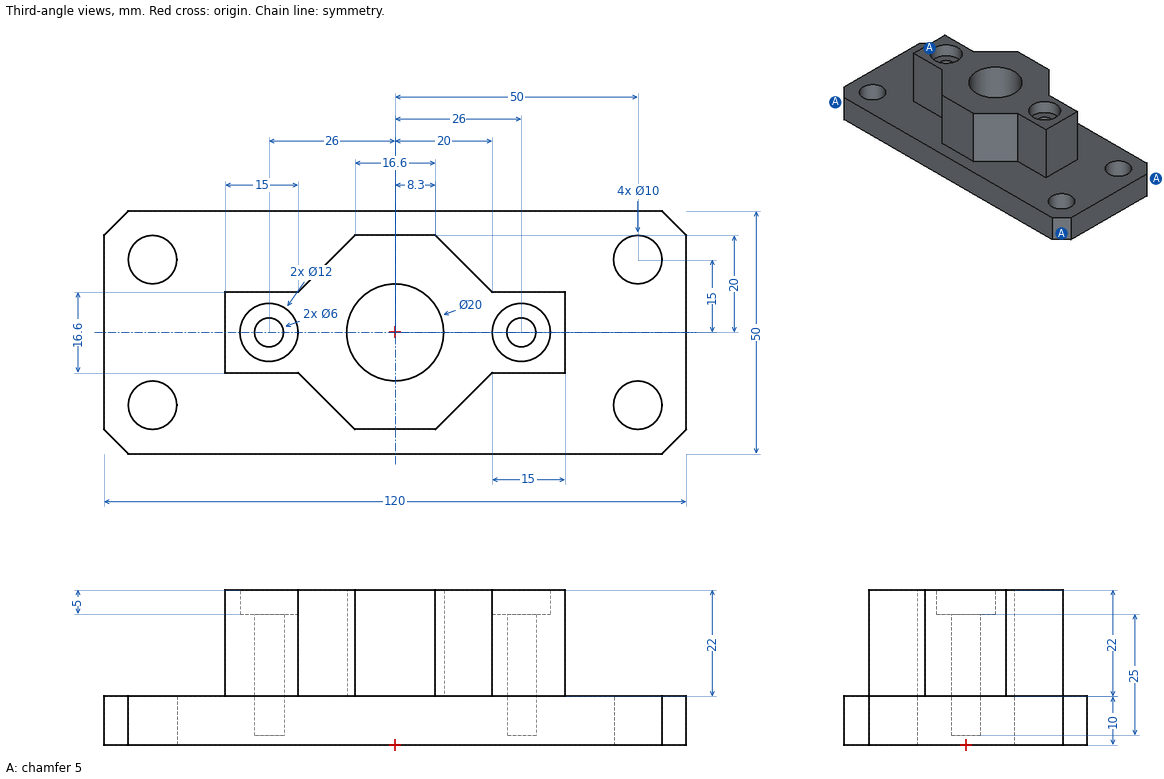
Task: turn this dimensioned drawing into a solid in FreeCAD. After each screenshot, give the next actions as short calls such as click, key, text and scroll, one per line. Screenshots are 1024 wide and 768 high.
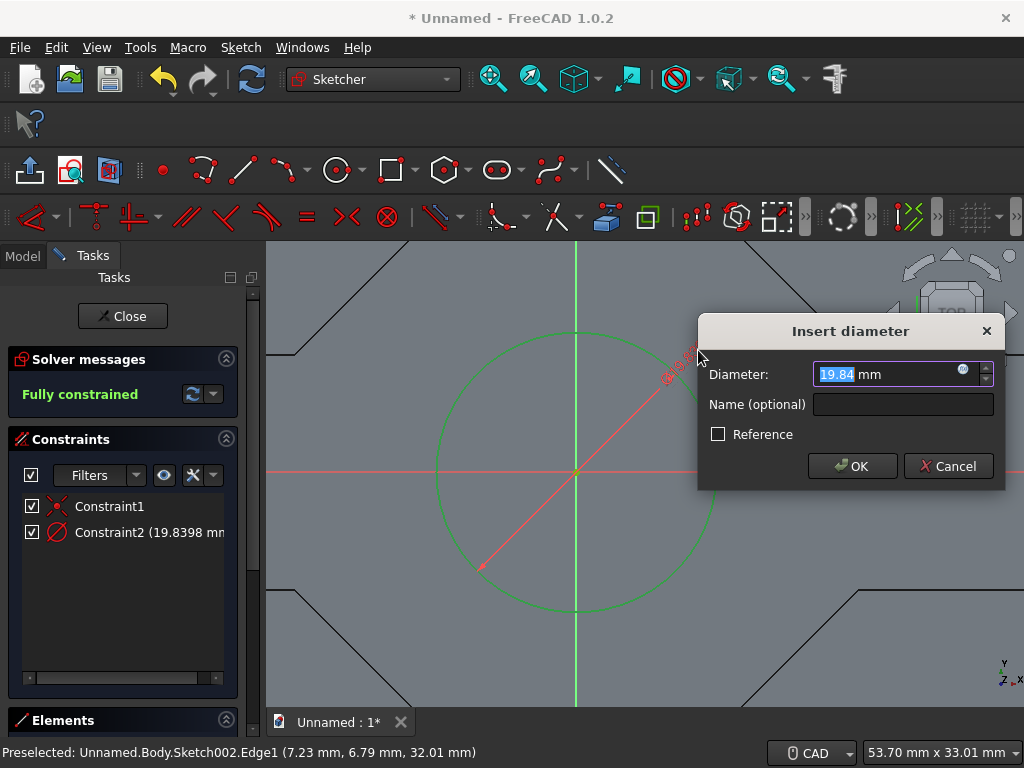
text(20)
key(Return)
key(Escape)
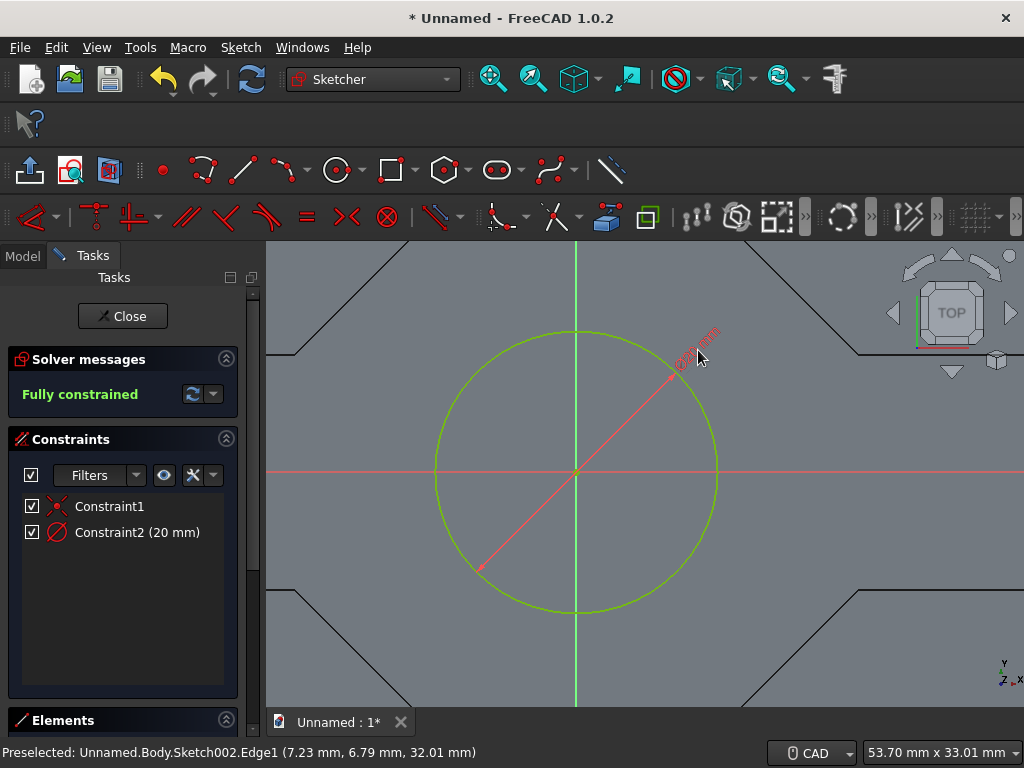
click(123, 316)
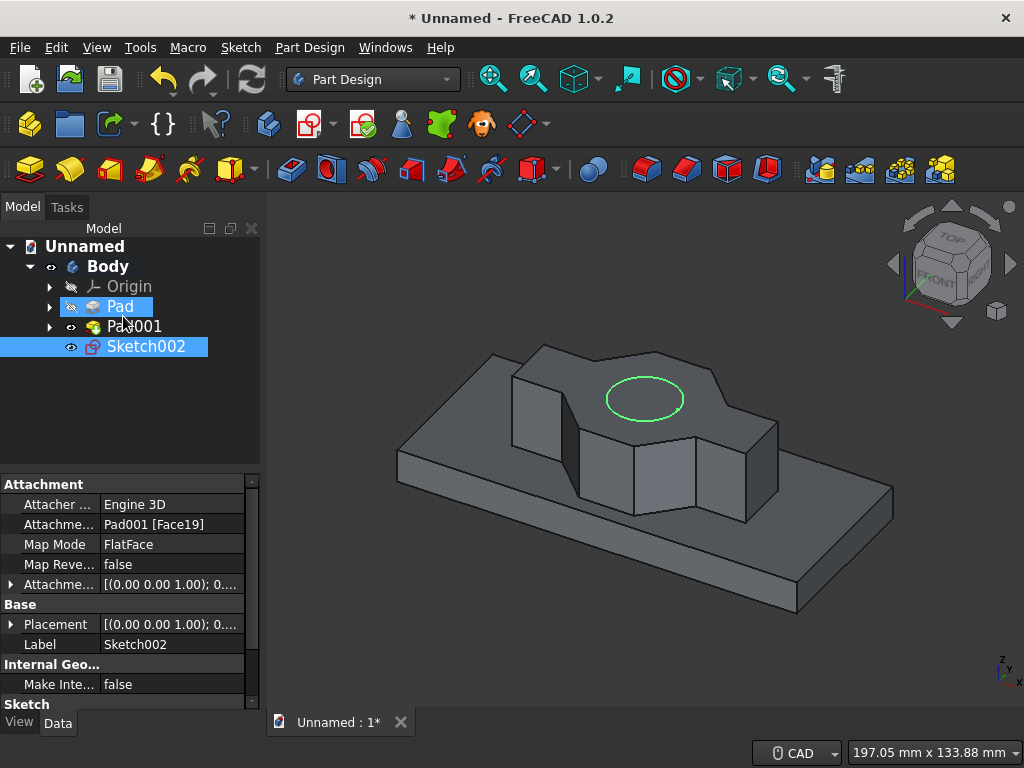
click(292, 170)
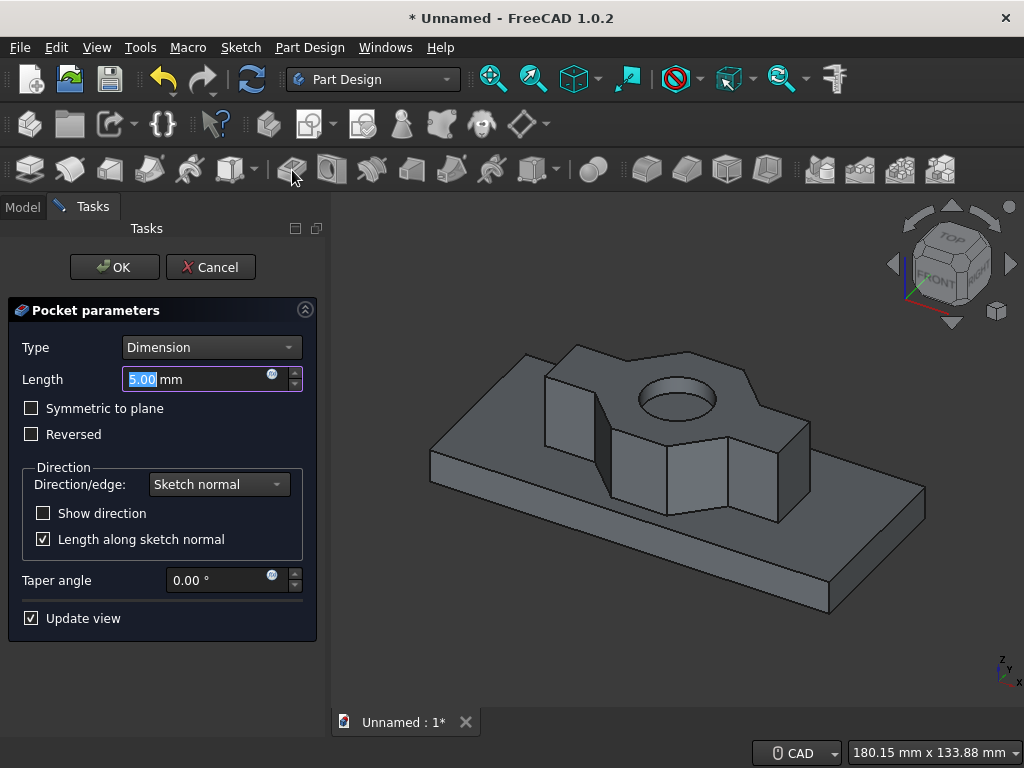
text(22)
key(Tab)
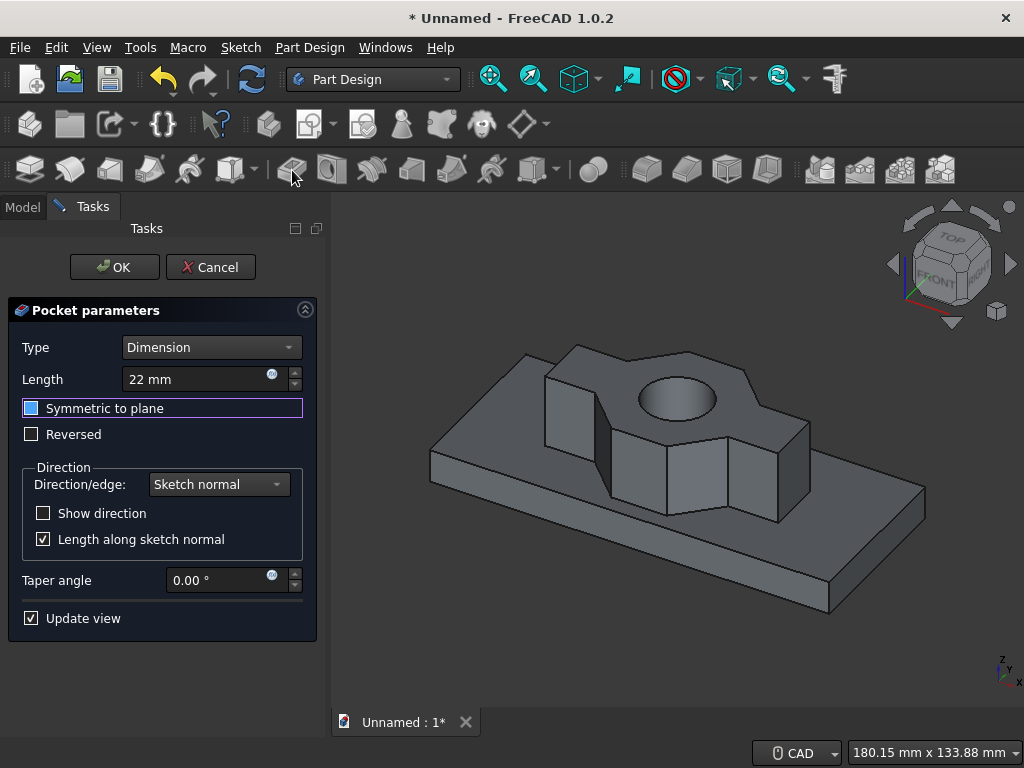
click(115, 267)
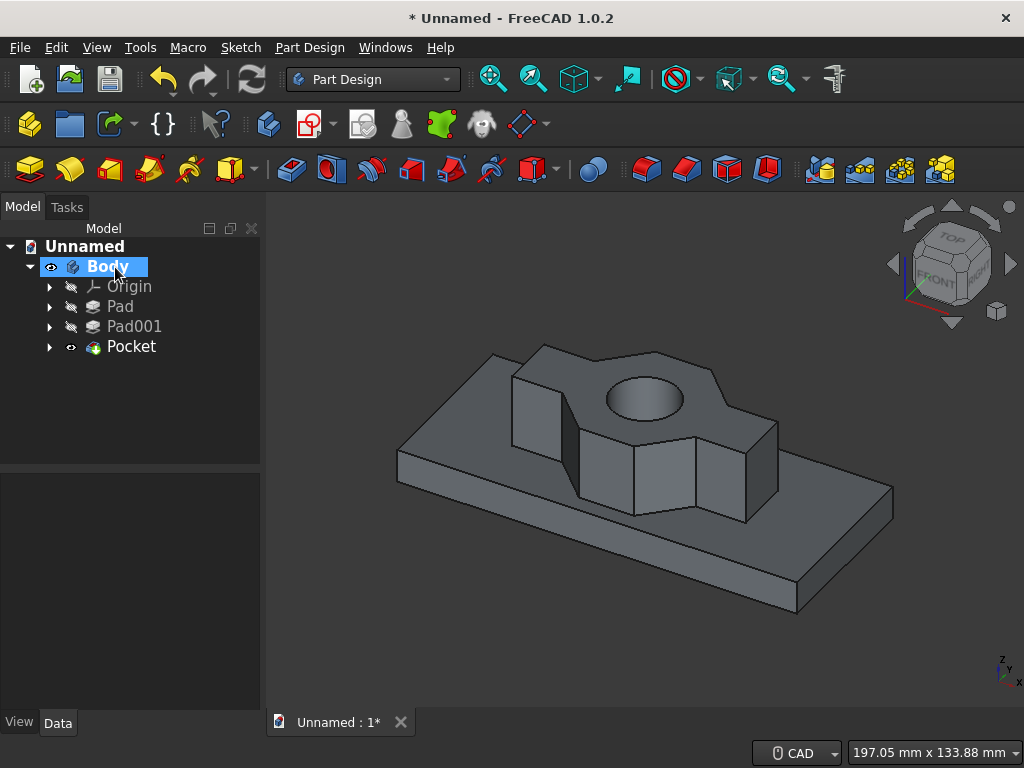
click(712, 420)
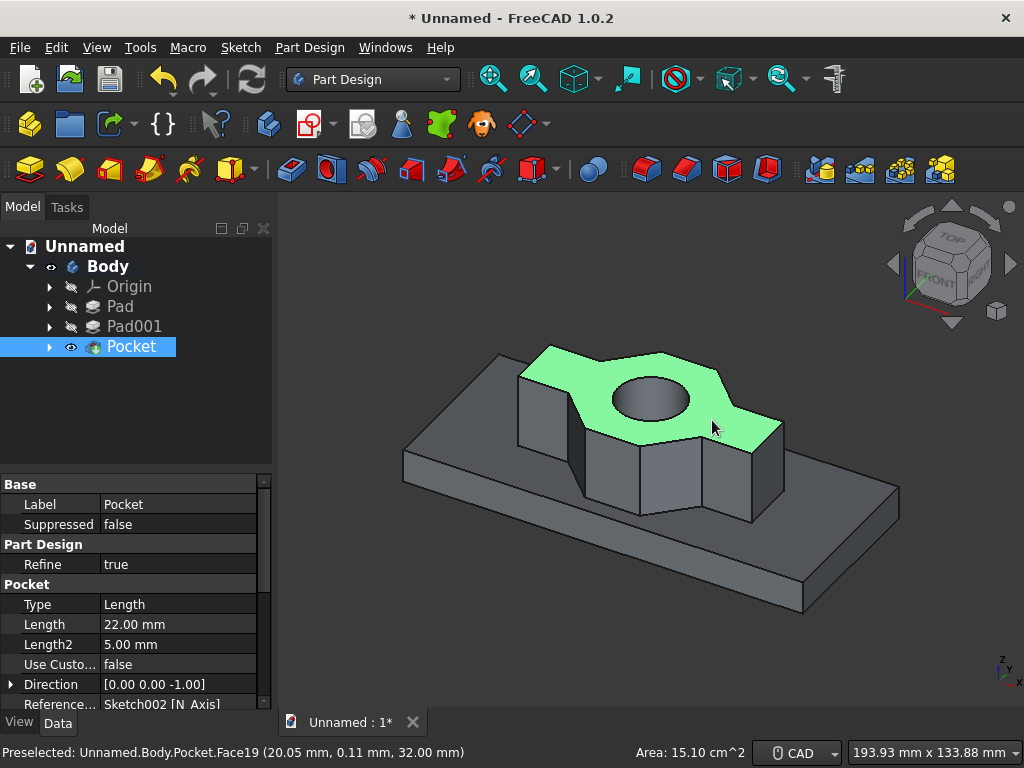
click(310, 124)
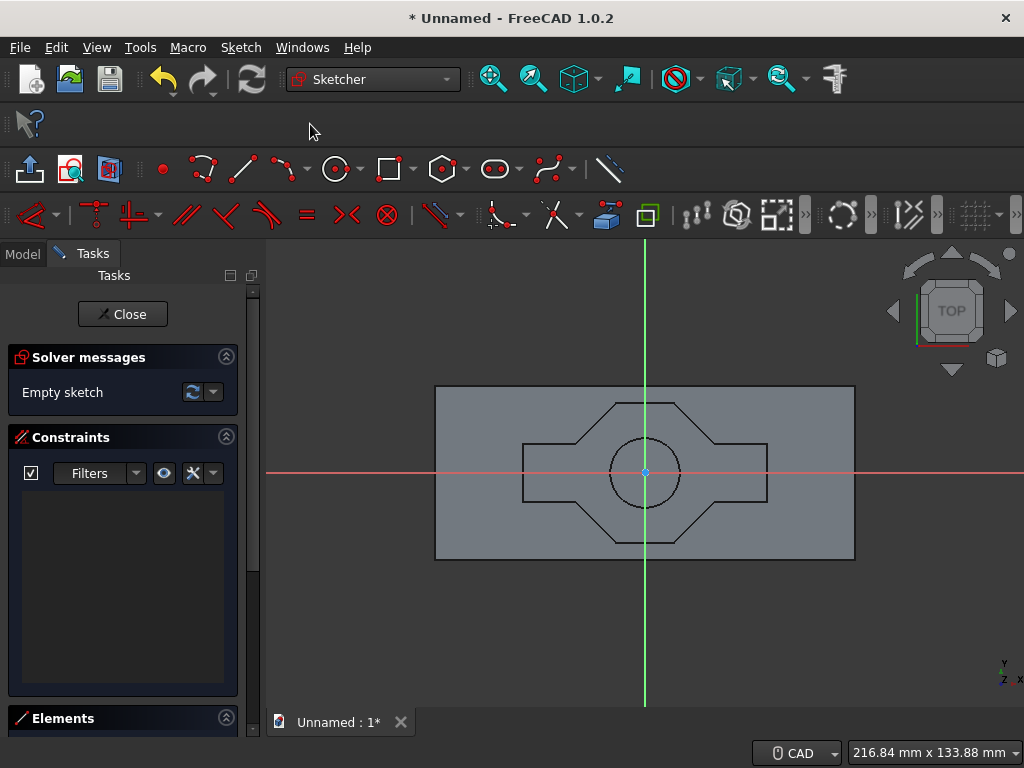
scroll(728, 473, up, 3)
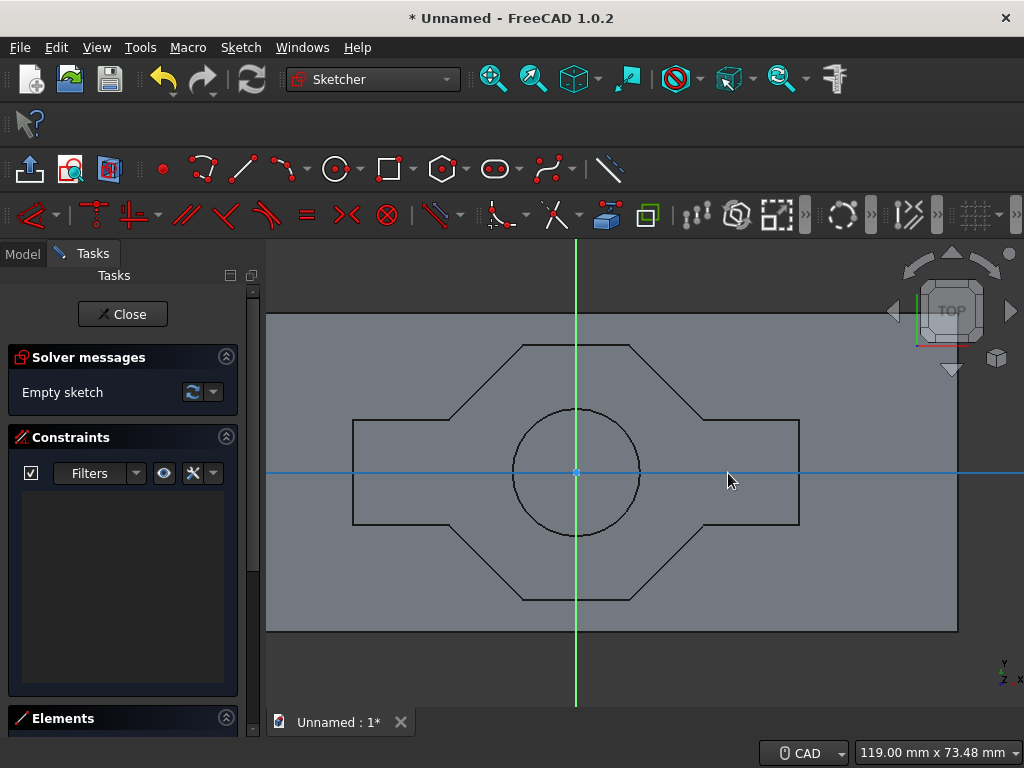
click(336, 170)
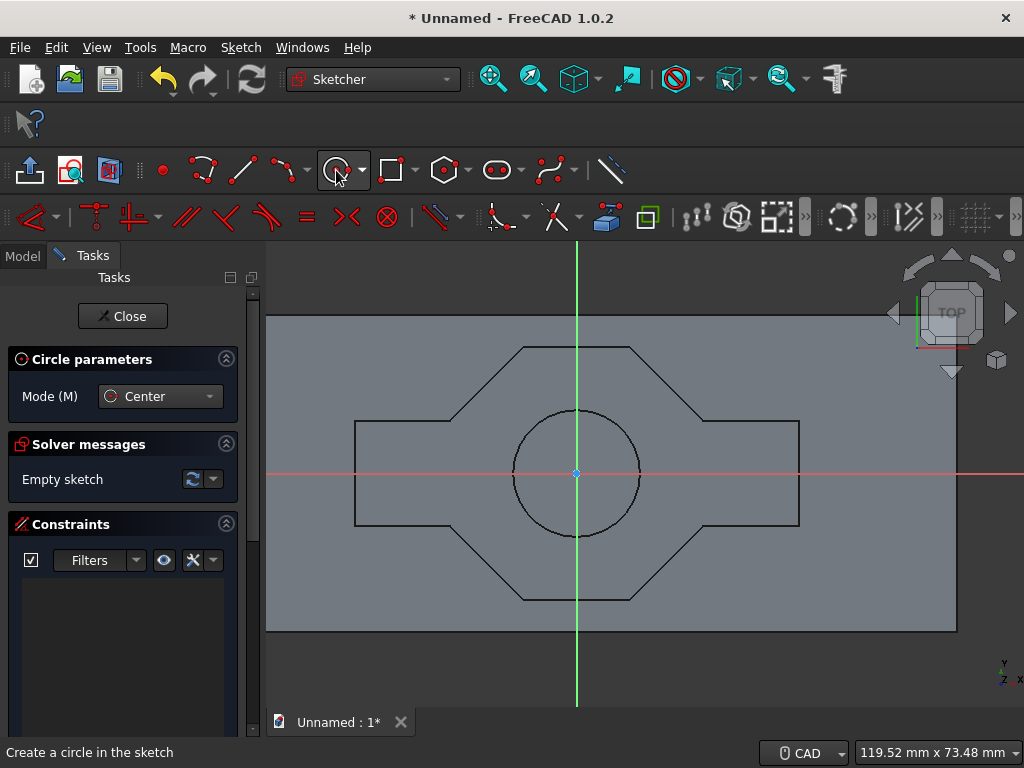
click(412, 474)
click(439, 447)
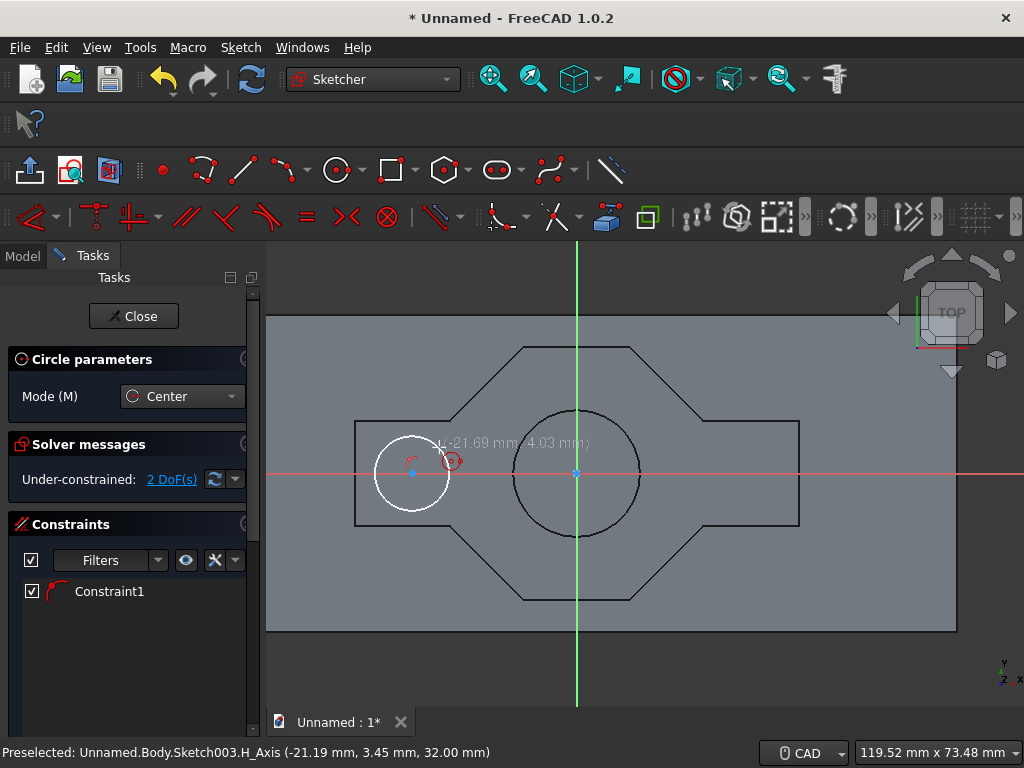
click(741, 474)
click(768, 447)
key(Escape)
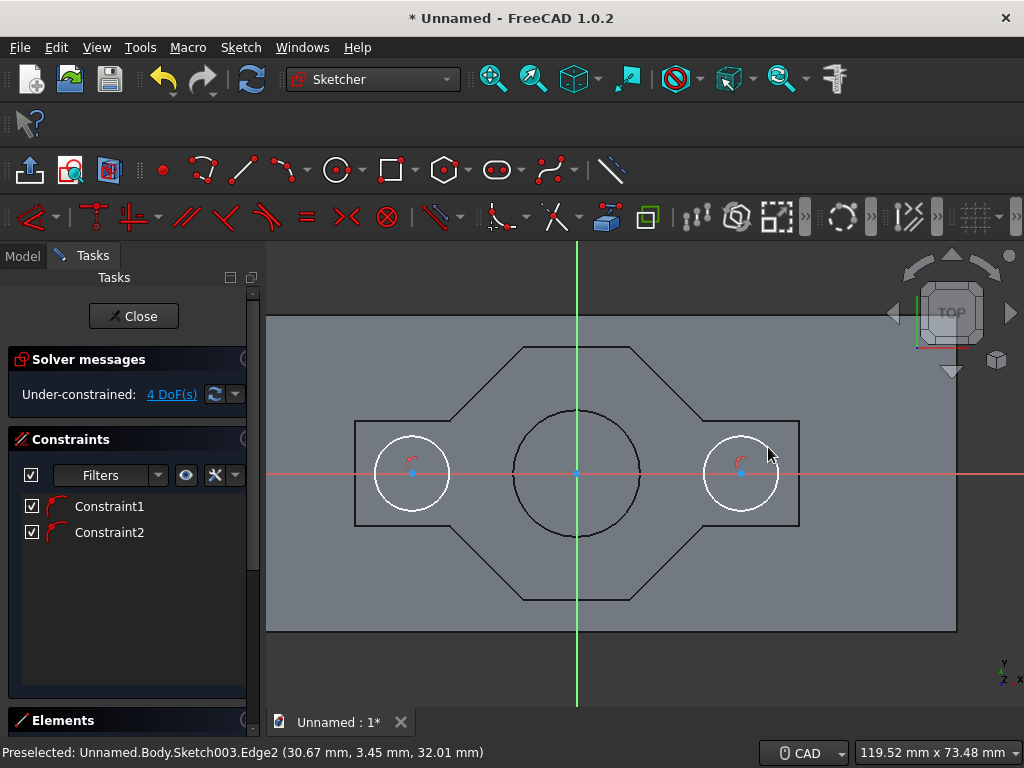
click(438, 447)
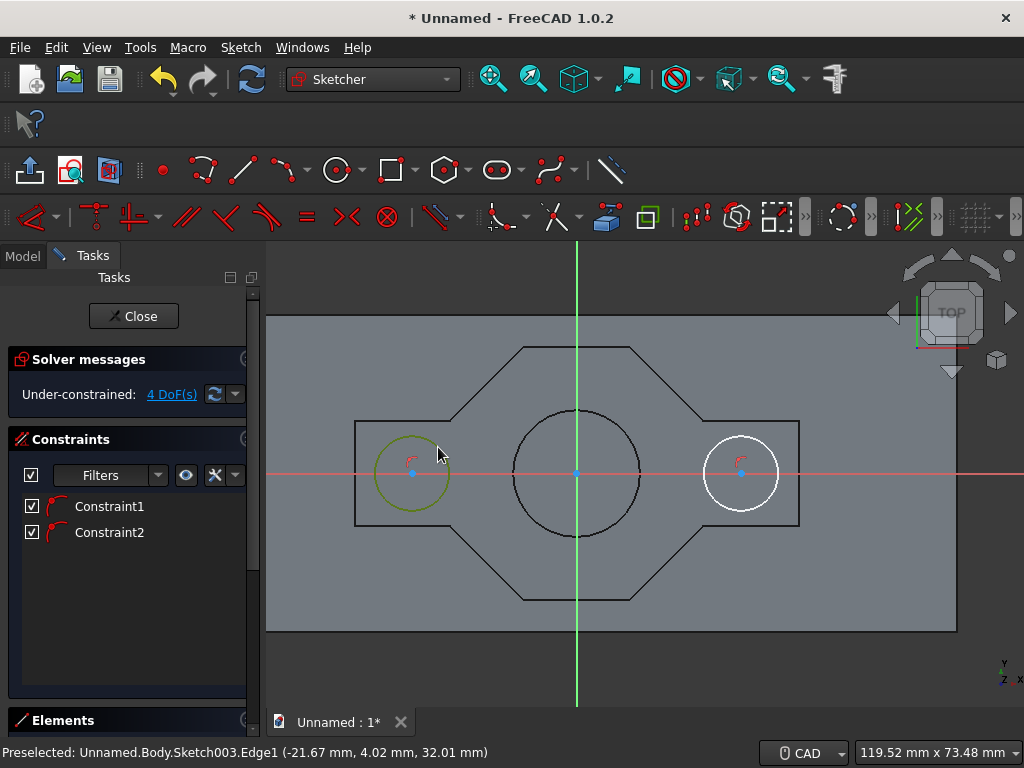
click(767, 447)